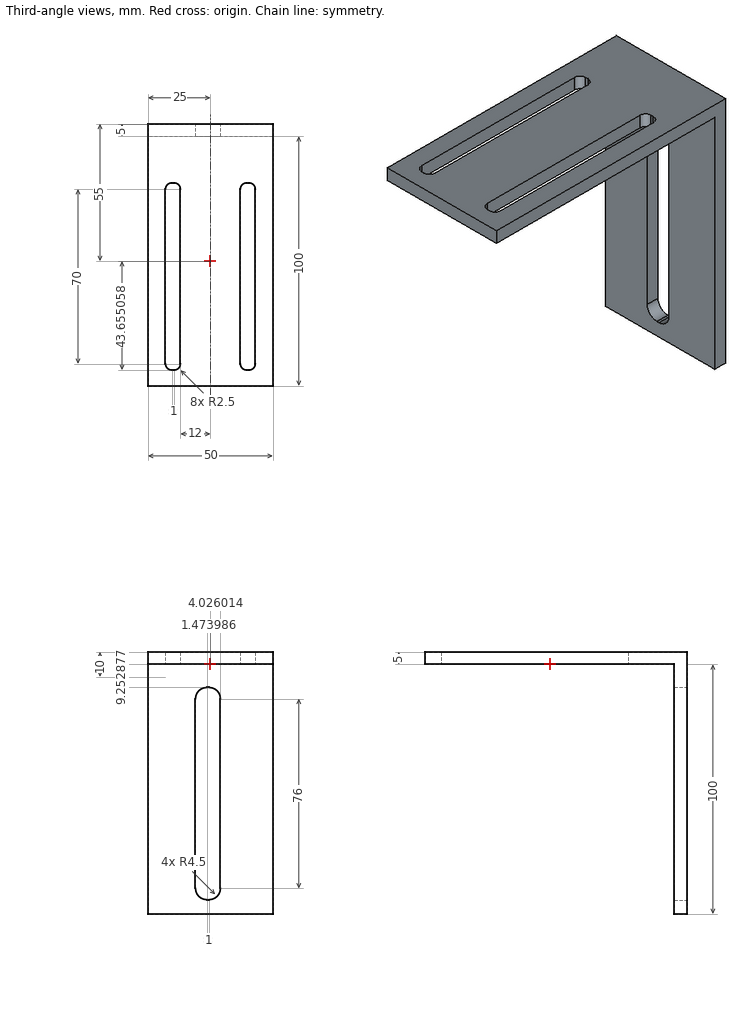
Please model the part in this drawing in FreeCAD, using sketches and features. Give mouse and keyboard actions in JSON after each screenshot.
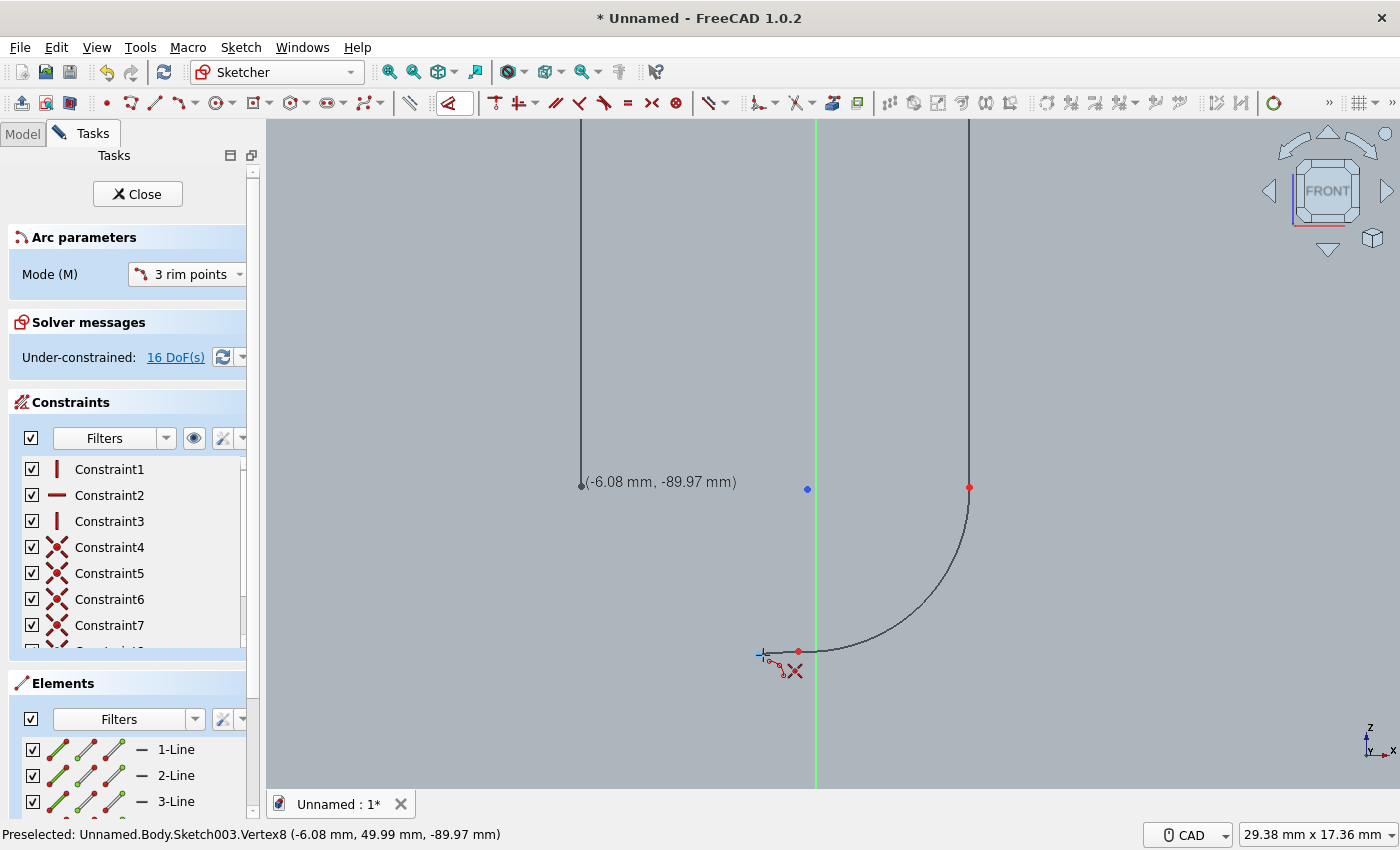
{"action": "left_click", "coordinate": [758, 654]}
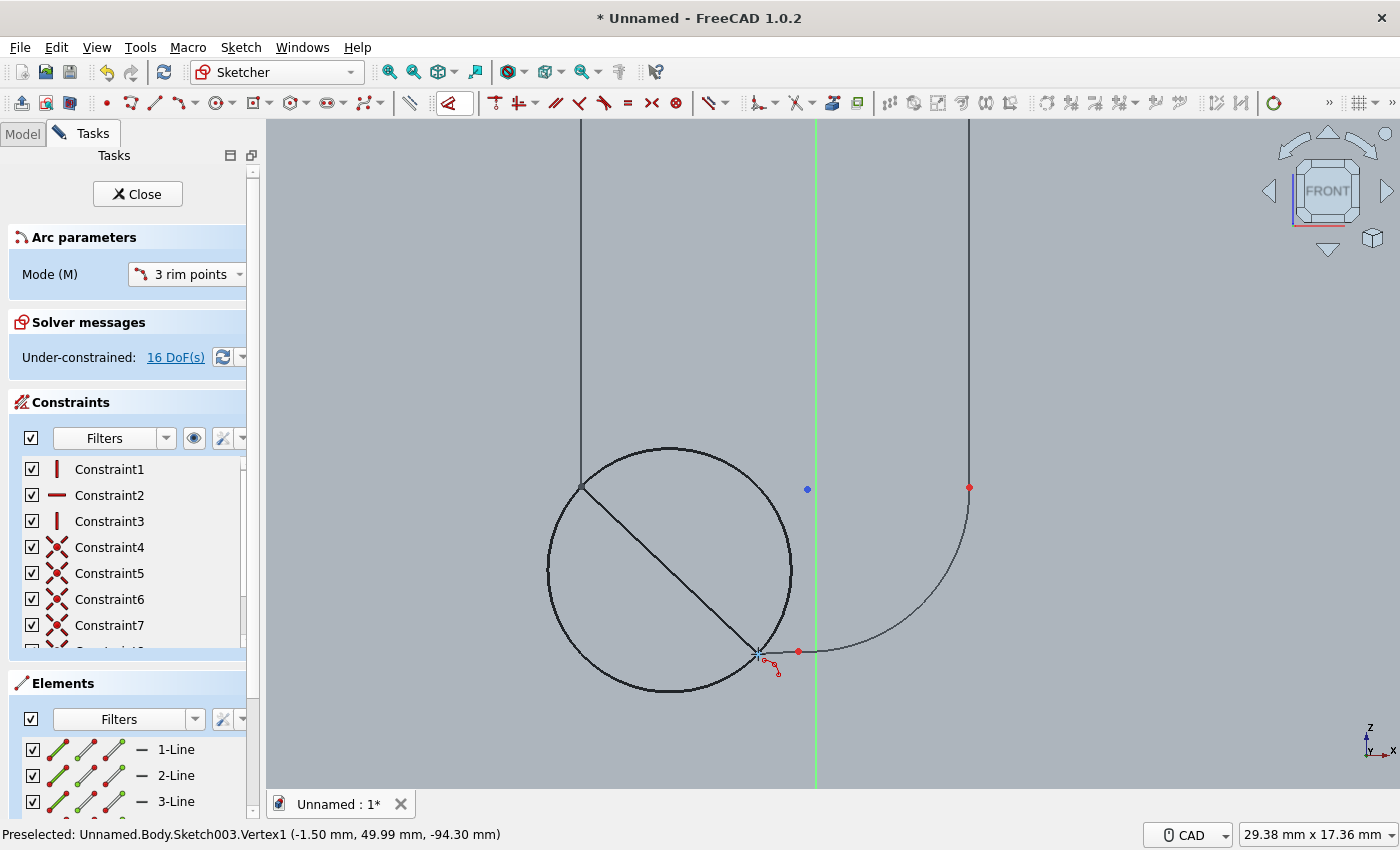
{"action": "scroll", "coordinate": [763, 656], "scroll_direction": "down", "scroll_amount": 11}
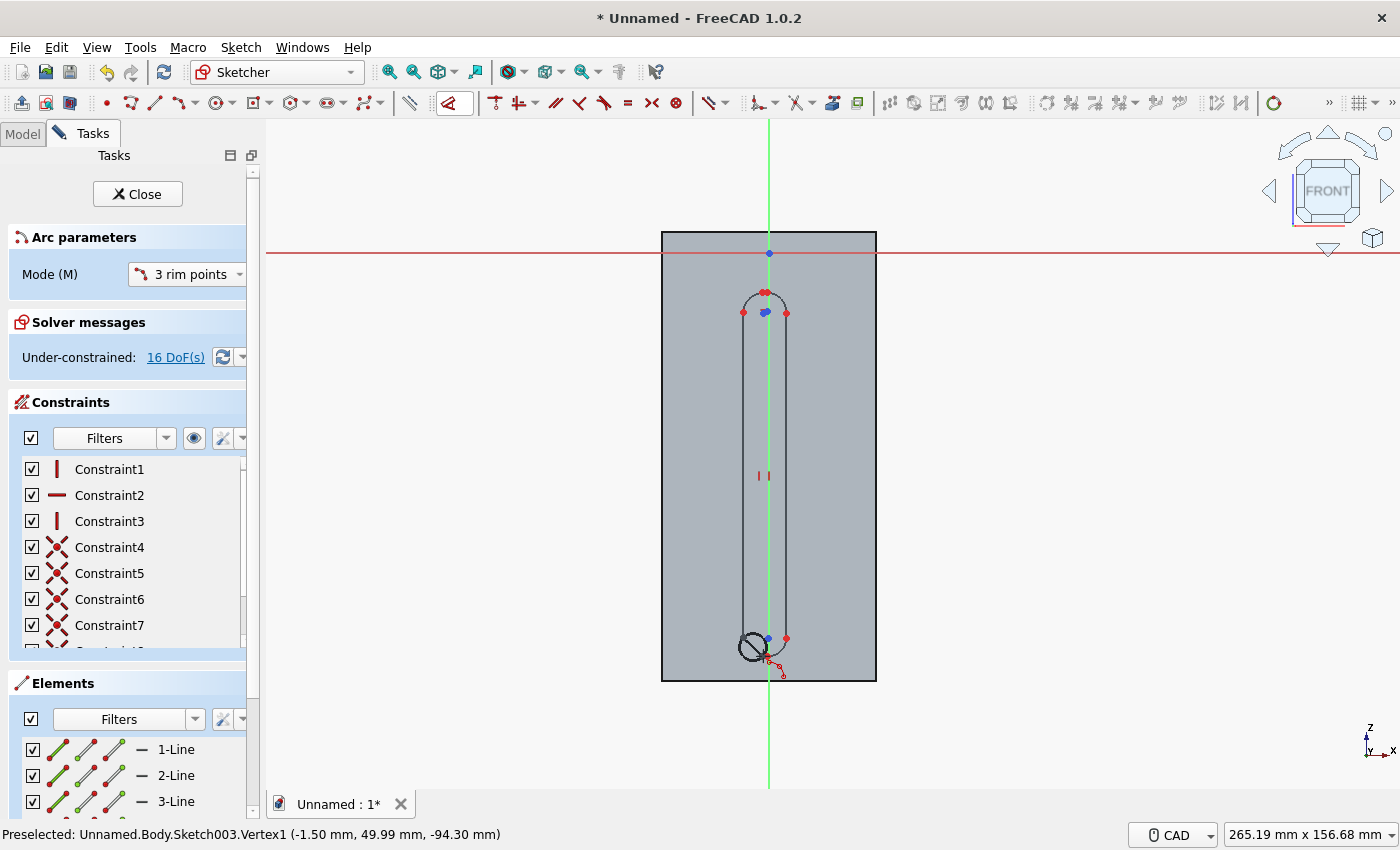
{"action": "scroll", "coordinate": [749, 651], "scroll_direction": "up", "scroll_amount": 6}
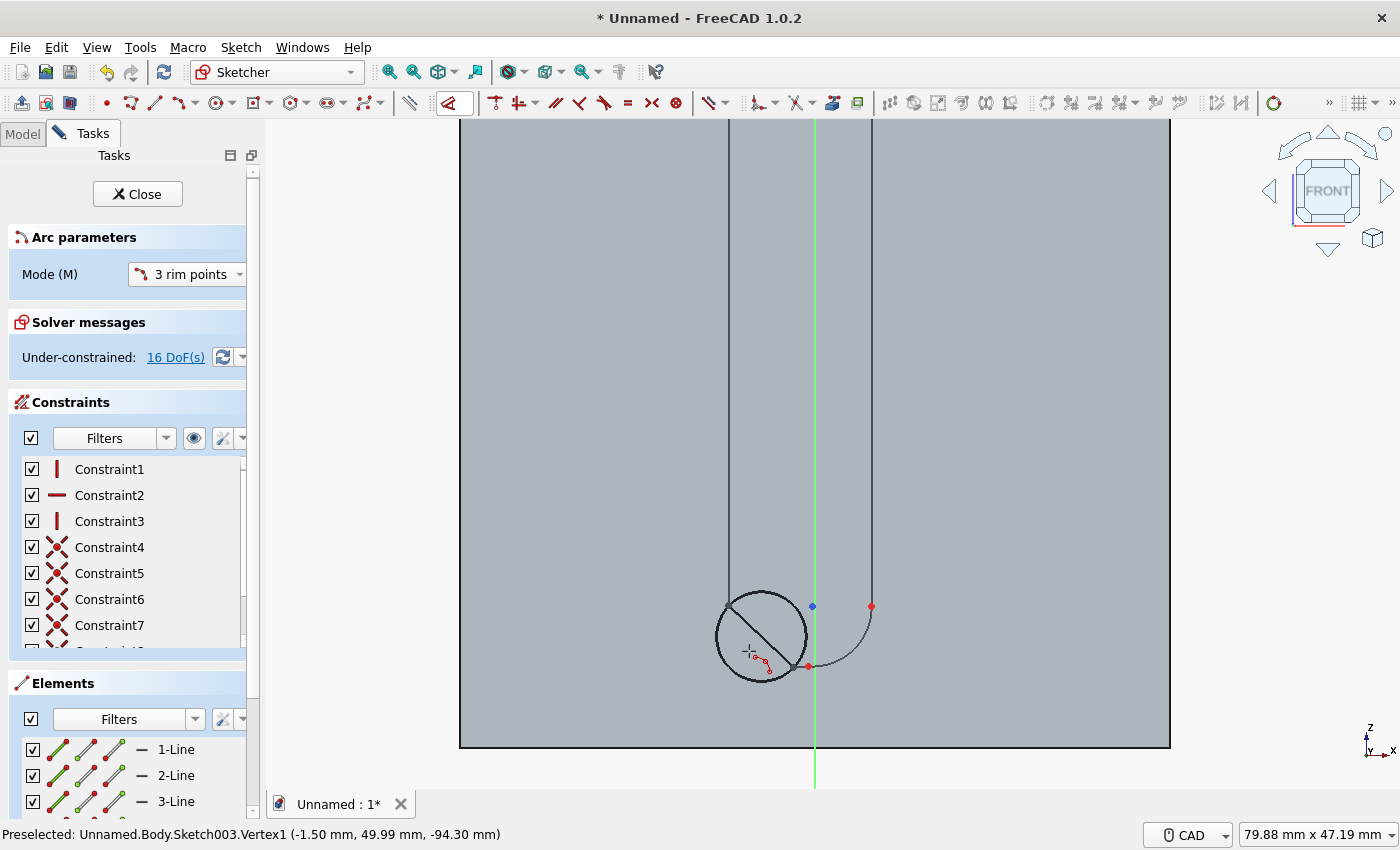
{"action": "left_click", "coordinate": [749, 648]}
{"action": "key", "text": "Escape"}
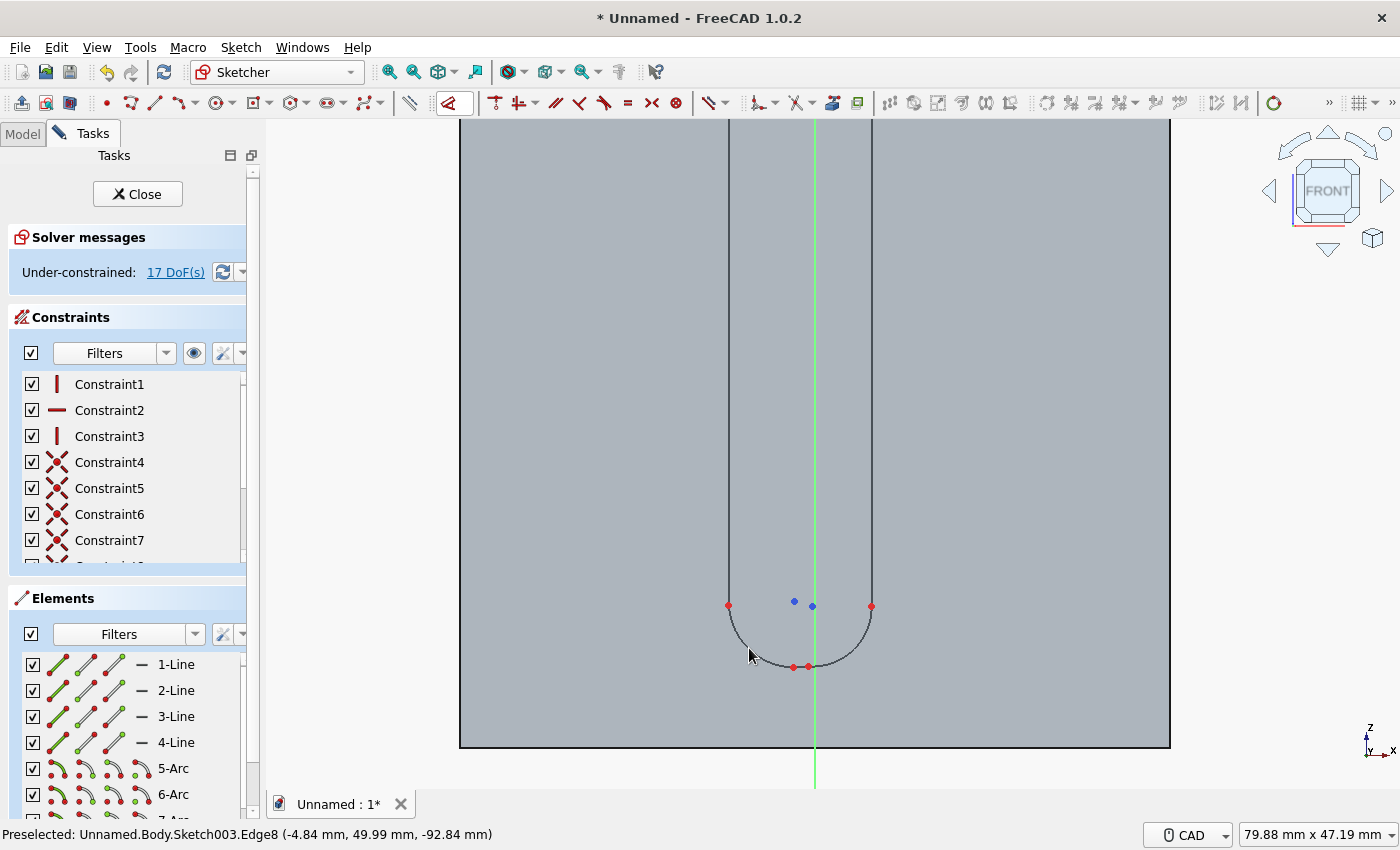
{"action": "scroll", "coordinate": [801, 667], "scroll_direction": "up", "scroll_amount": 4}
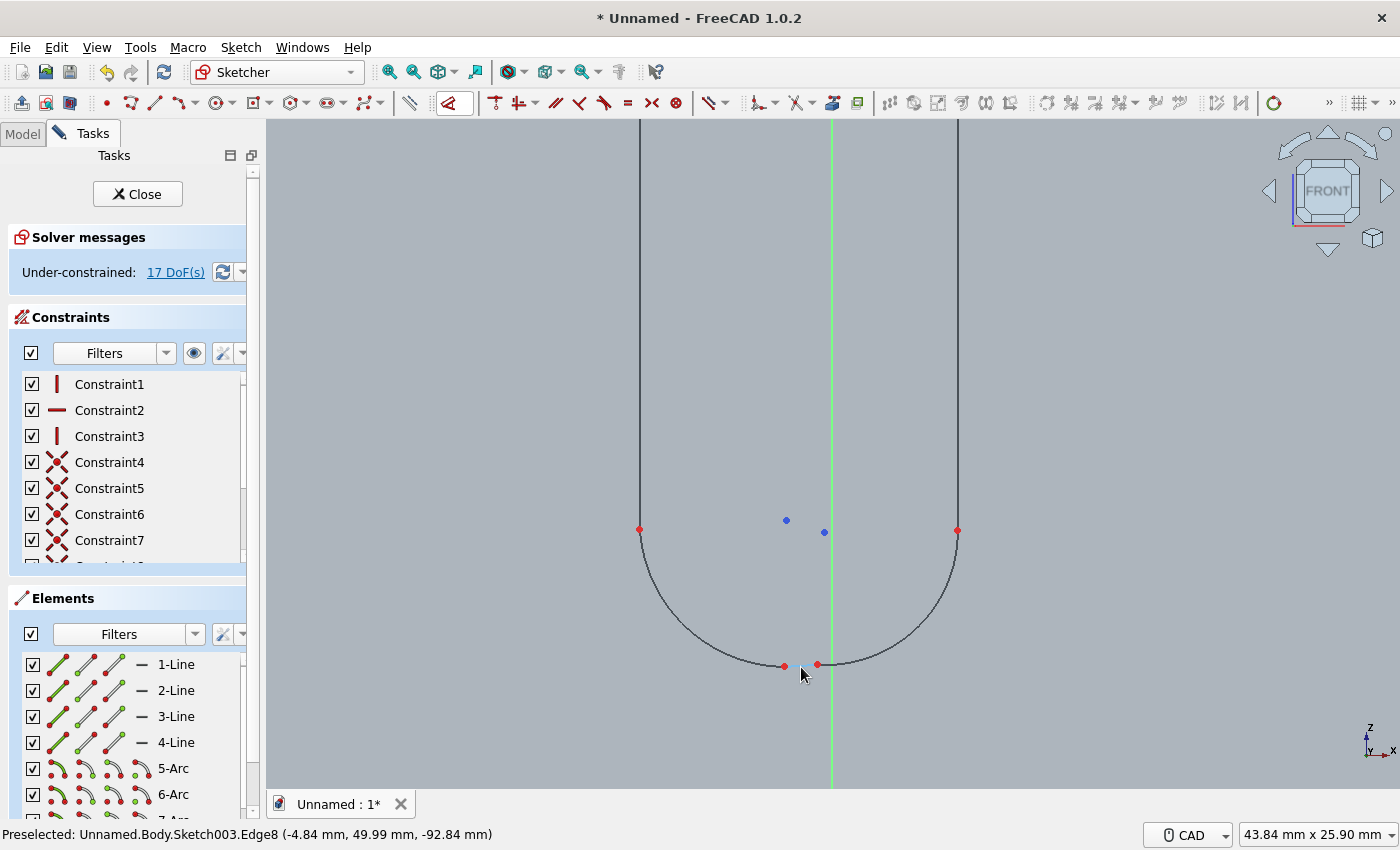
{"action": "left_click", "coordinate": [801, 666]}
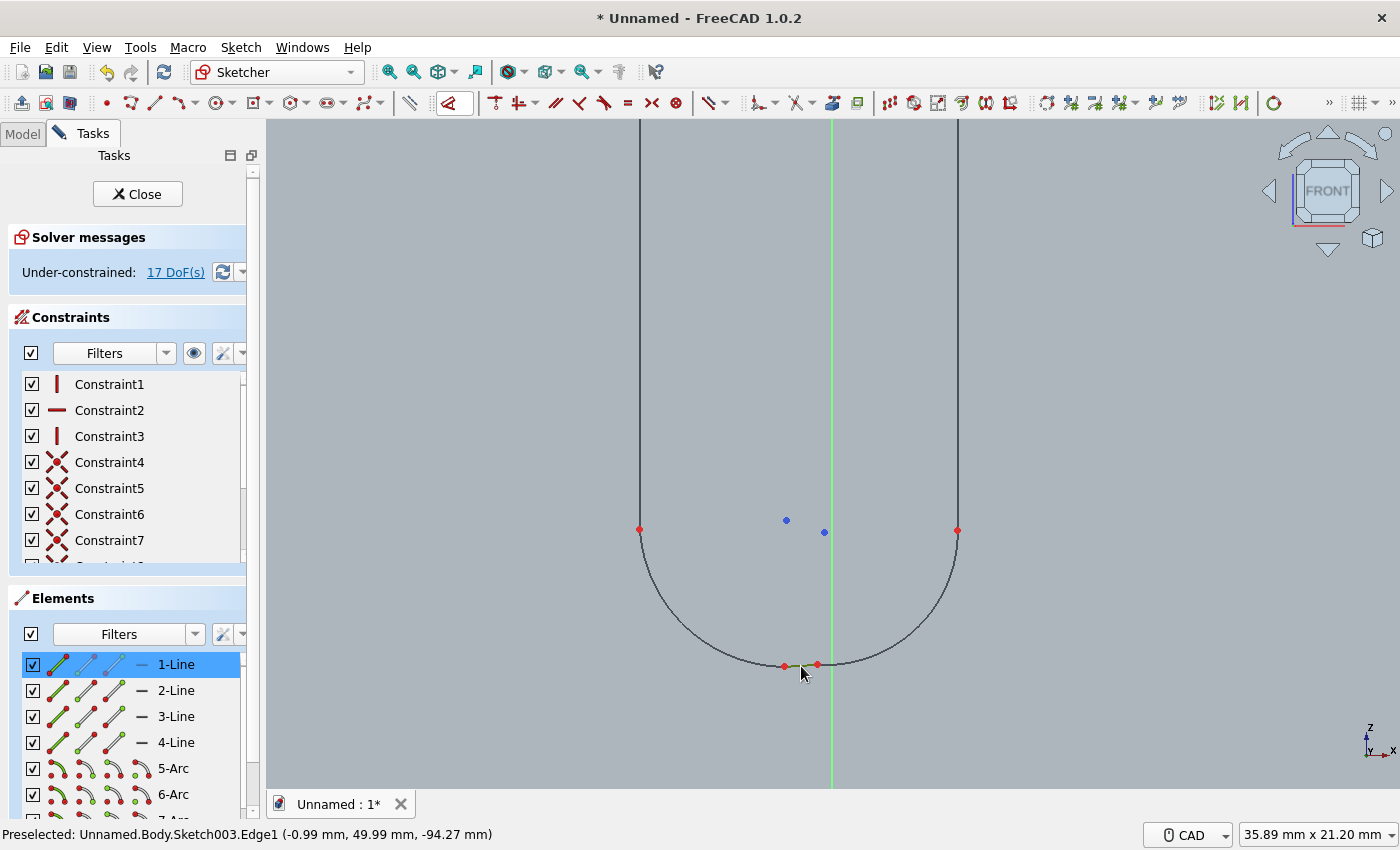
{"action": "scroll", "coordinate": [759, 654], "scroll_direction": "down", "scroll_amount": 10}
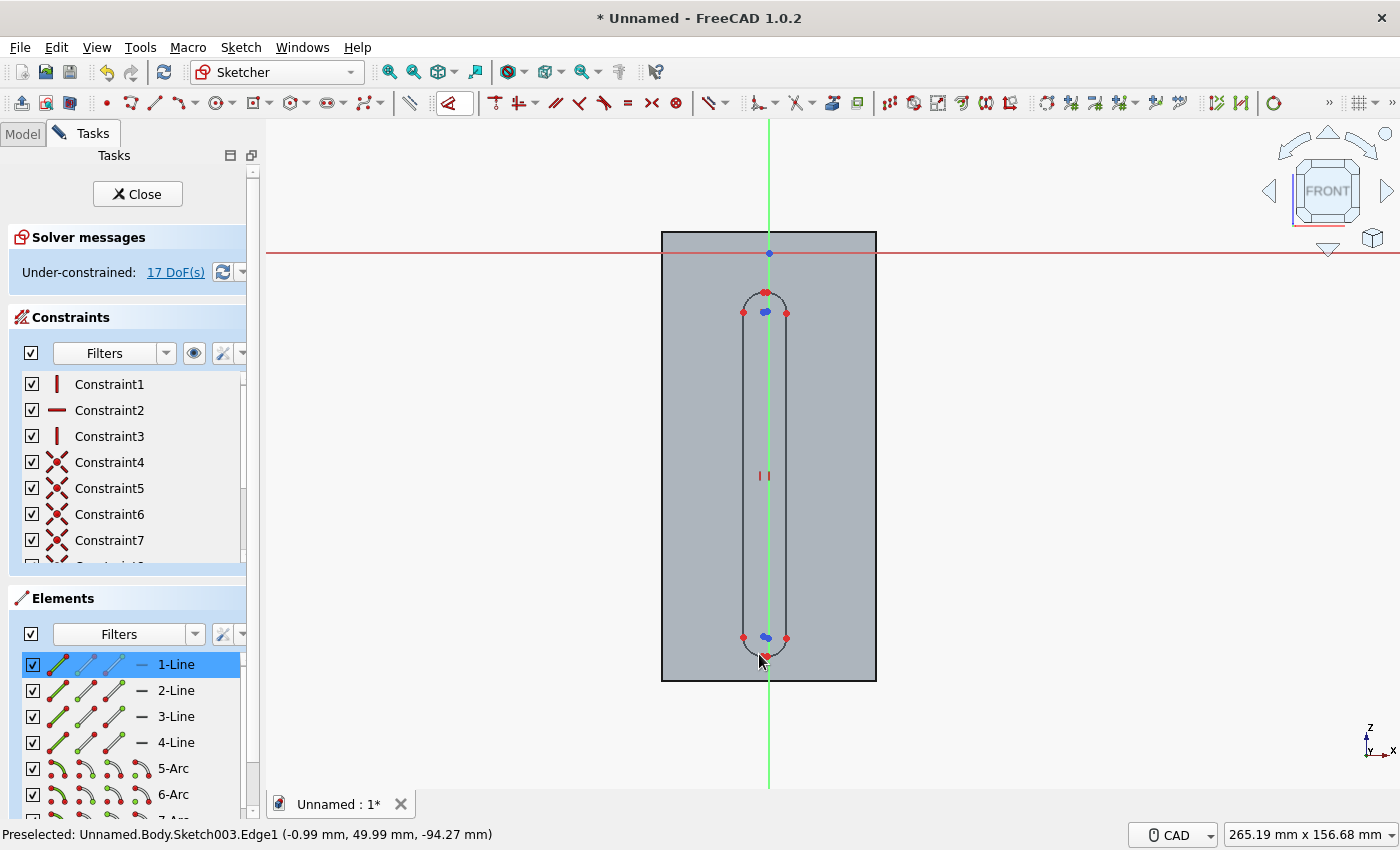
{"action": "scroll", "coordinate": [776, 655], "scroll_direction": "up", "scroll_amount": 4}